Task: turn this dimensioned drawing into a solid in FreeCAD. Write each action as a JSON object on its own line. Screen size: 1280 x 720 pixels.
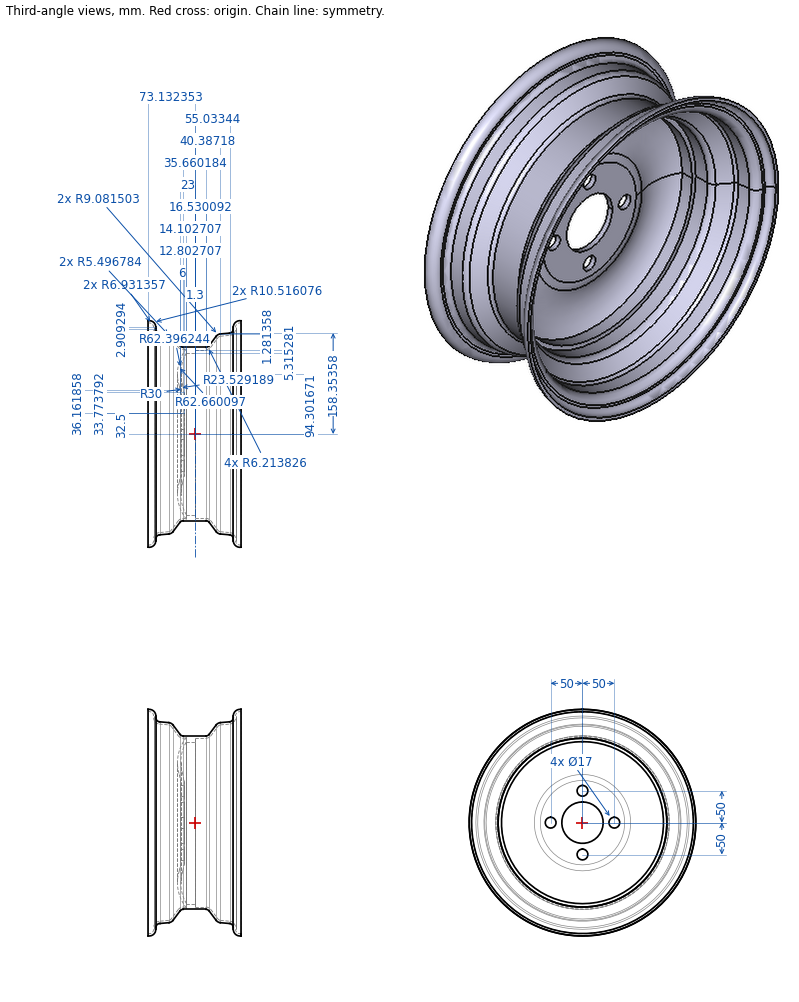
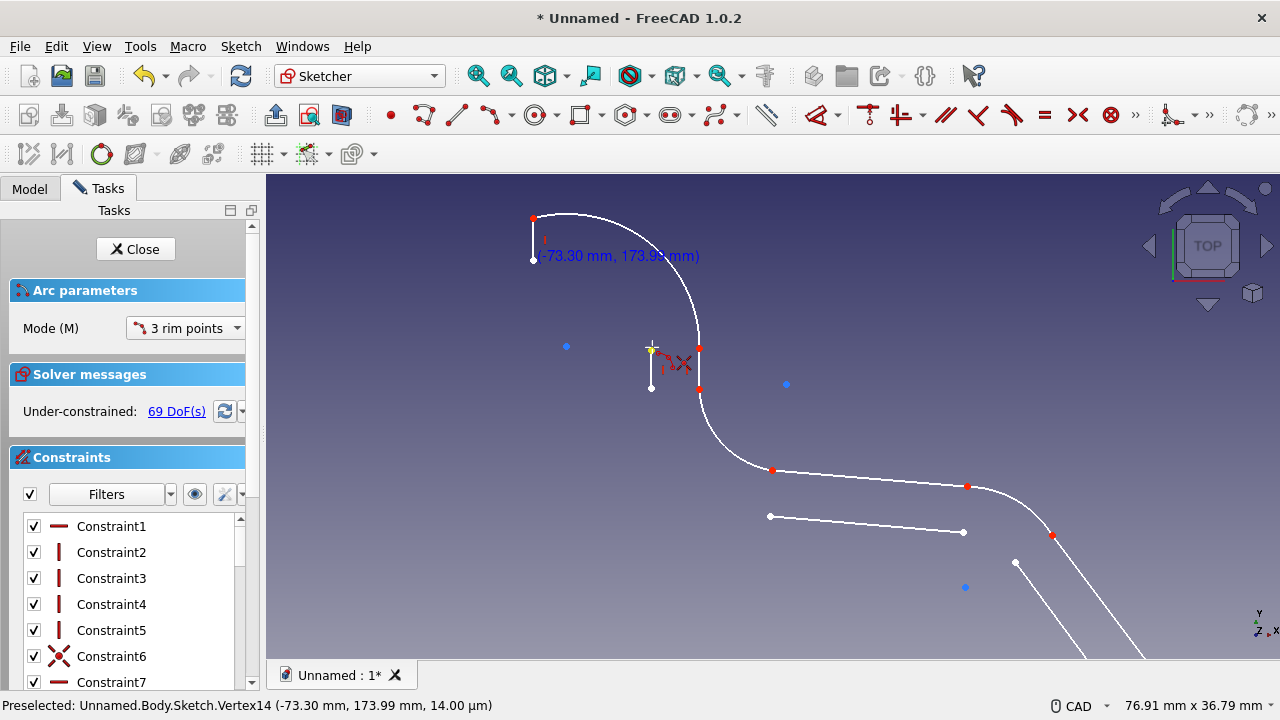
{"action": "left_click", "coordinate": [651, 351]}
{"action": "left_click", "coordinate": [615, 274]}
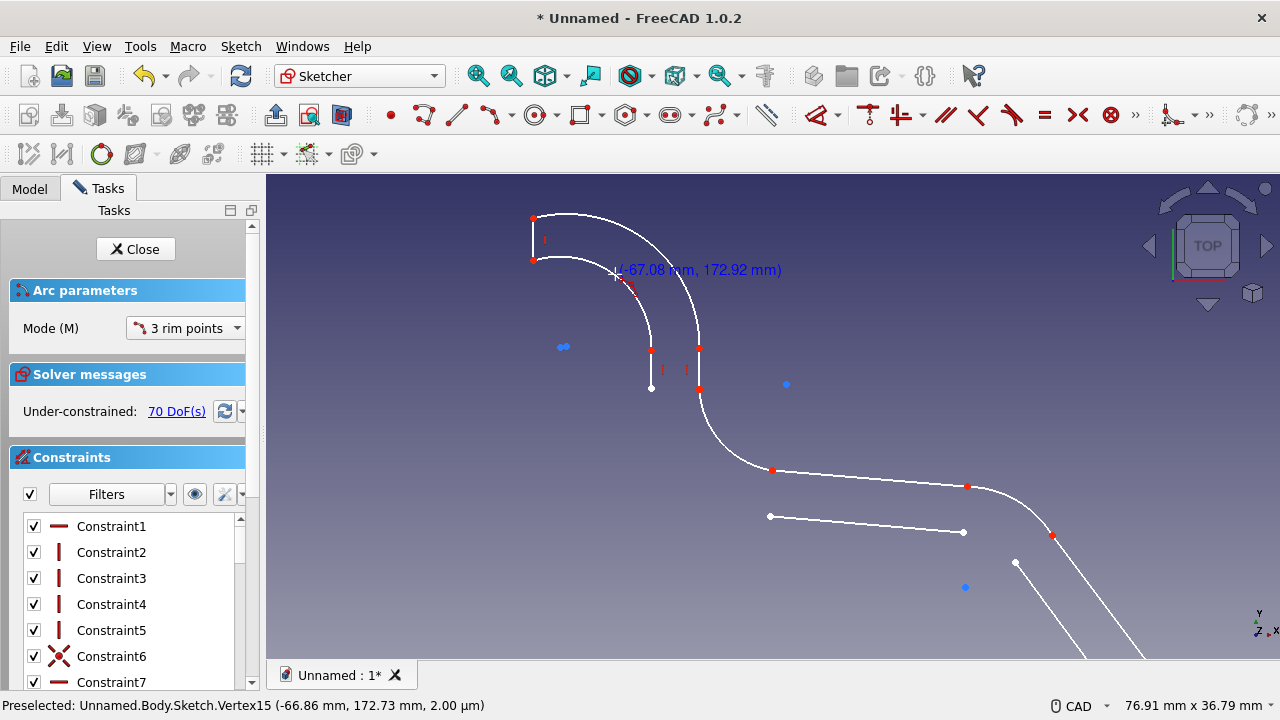
{"action": "left_click", "coordinate": [651, 389]}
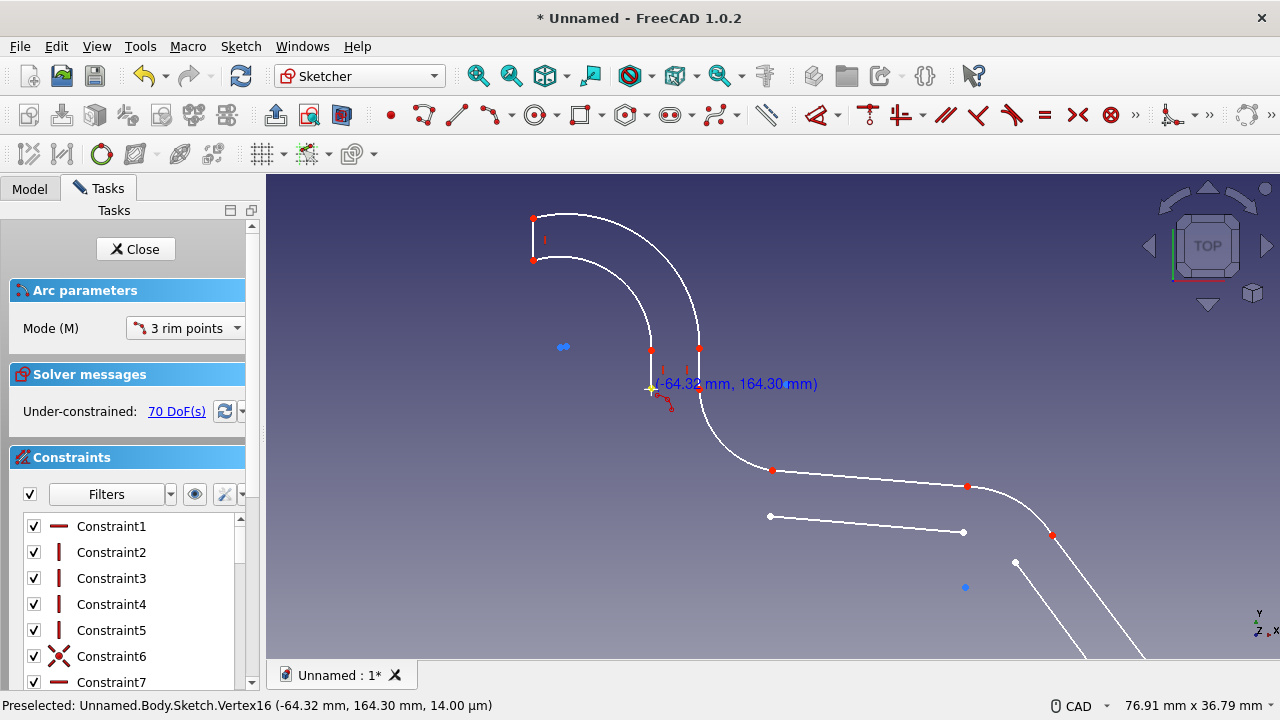
{"action": "scroll", "coordinate": [580, 265], "scroll_direction": "down", "scroll_amount": 10}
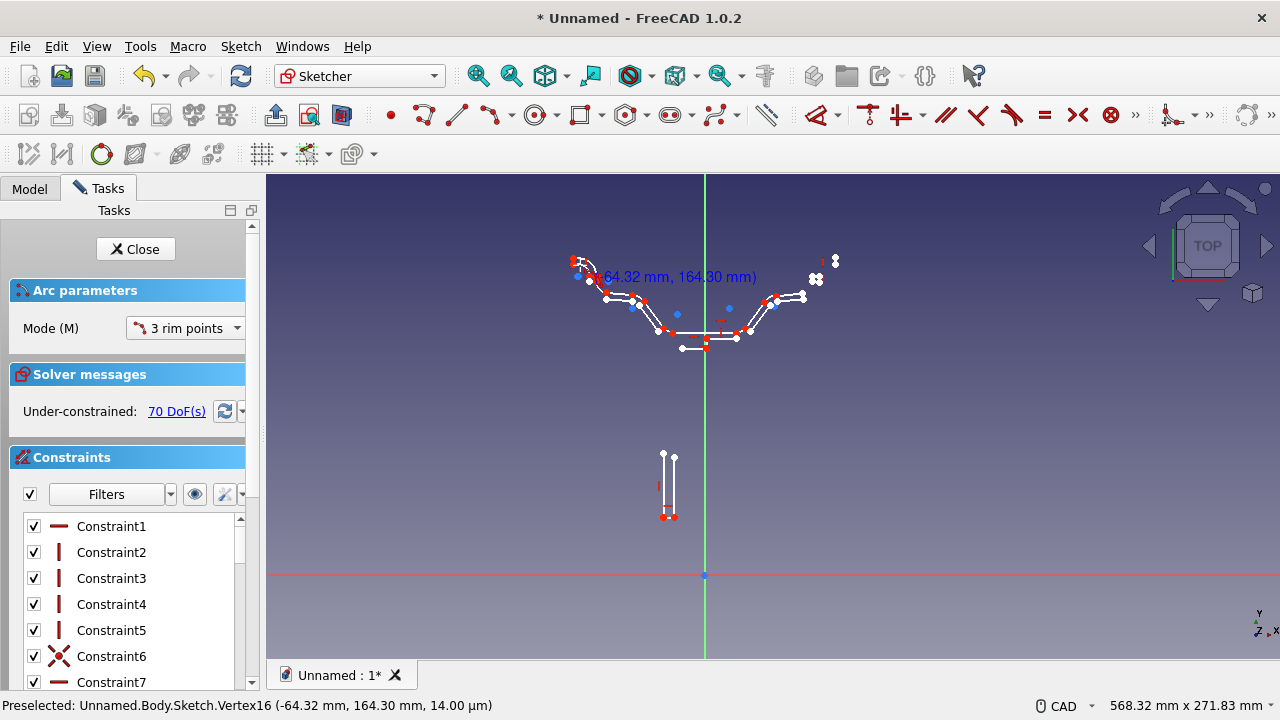
{"action": "scroll", "coordinate": [606, 299], "scroll_direction": "up", "scroll_amount": 5}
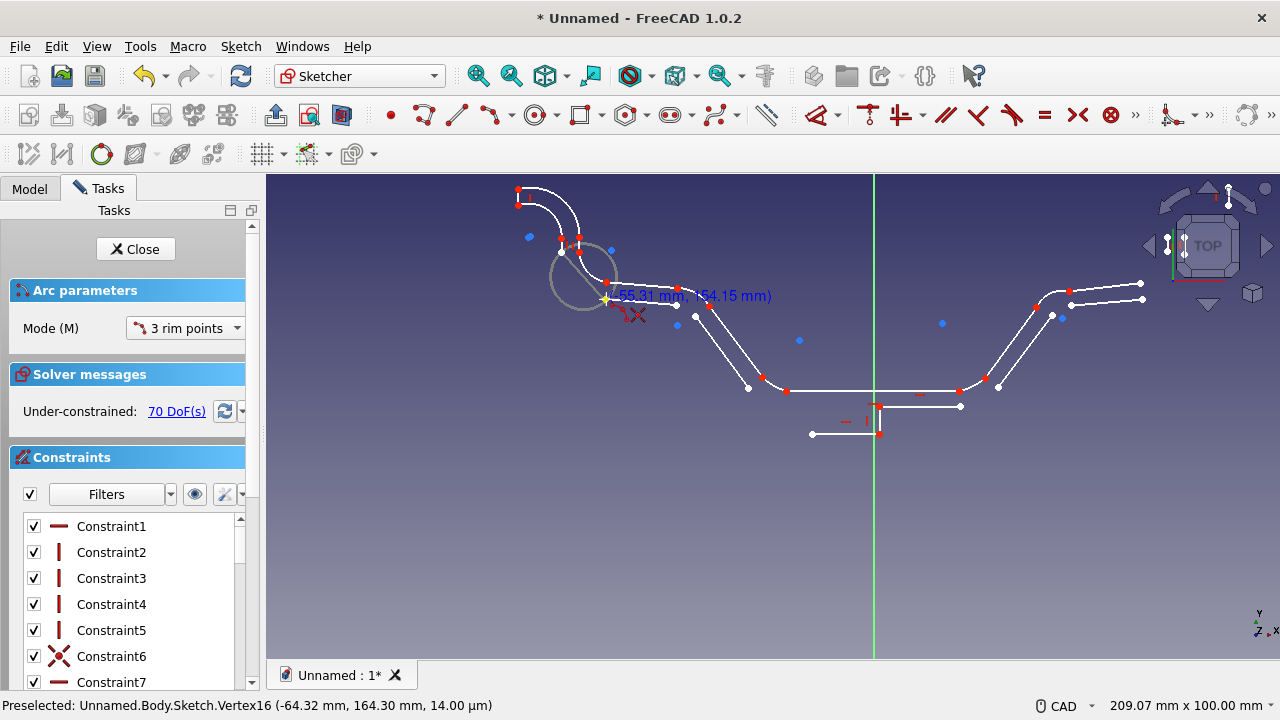
{"action": "left_click", "coordinate": [606, 299]}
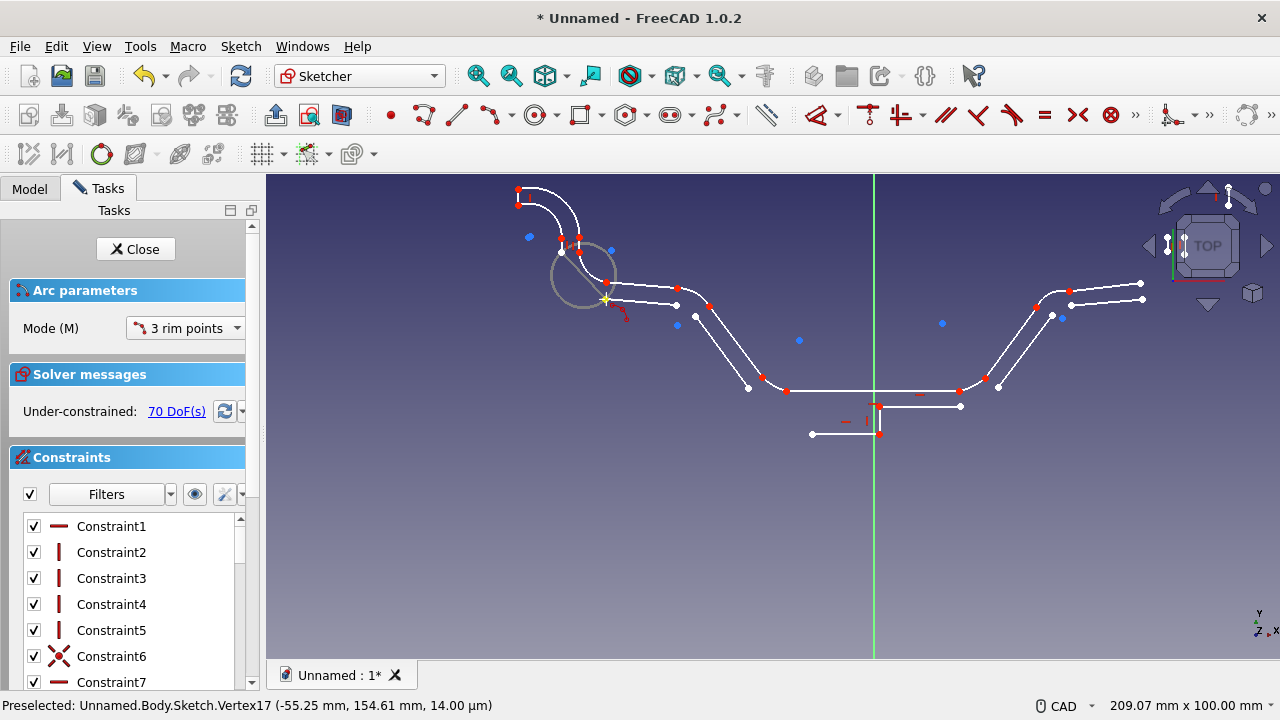
{"action": "scroll", "coordinate": [574, 283], "scroll_direction": "up", "scroll_amount": 2}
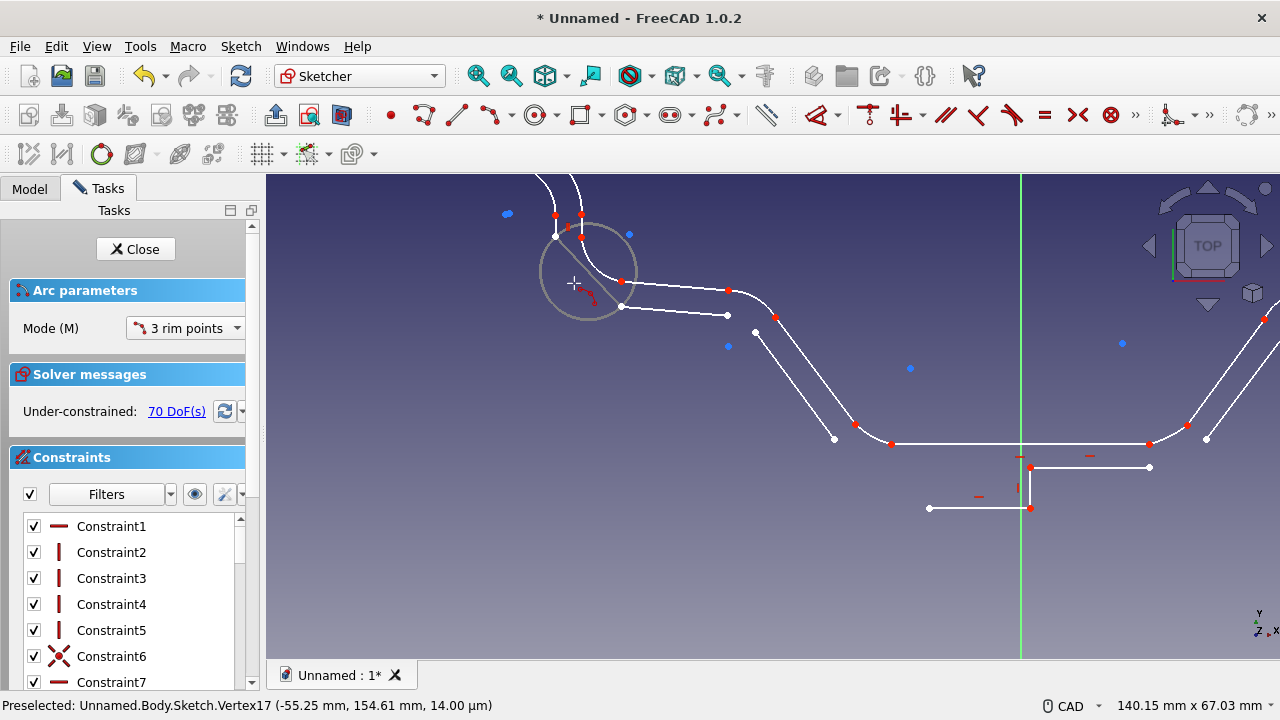
{"action": "left_click", "coordinate": [574, 283]}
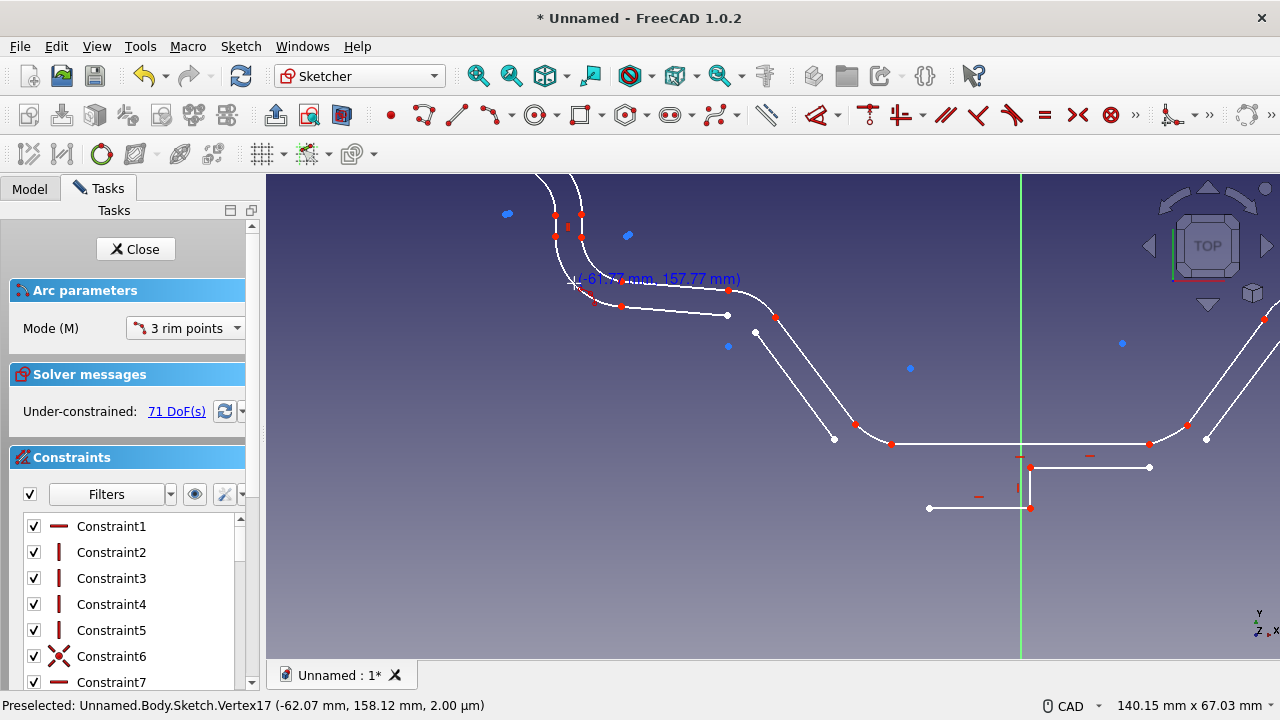
{"action": "left_click", "coordinate": [727, 316]}
{"action": "left_click", "coordinate": [755, 332]}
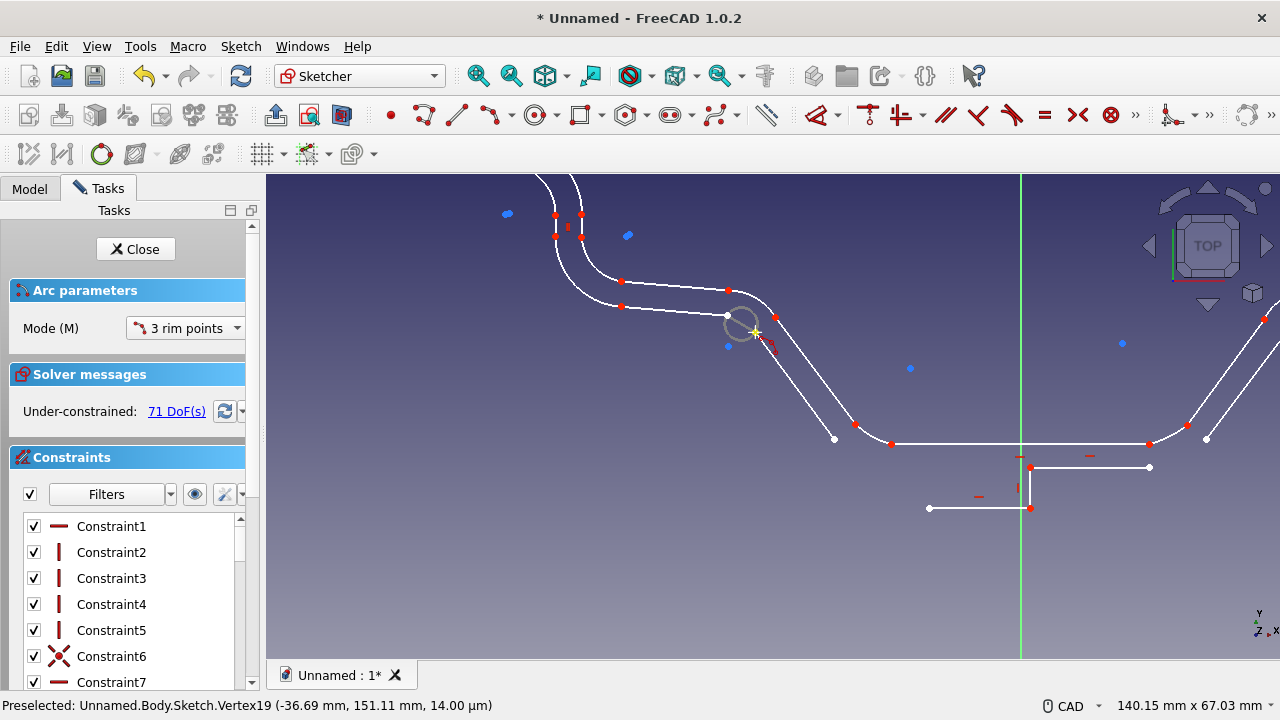
{"action": "scroll", "coordinate": [742, 320], "scroll_direction": "up", "scroll_amount": 8}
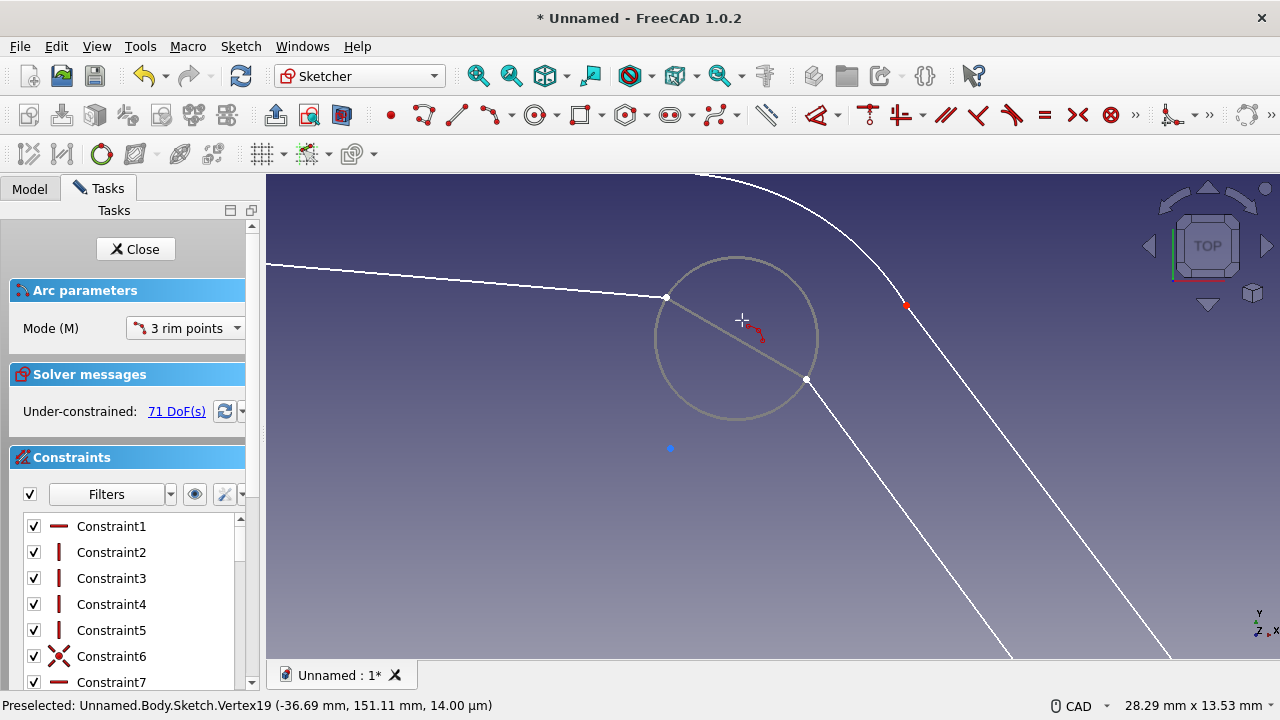
{"action": "left_click", "coordinate": [742, 318]}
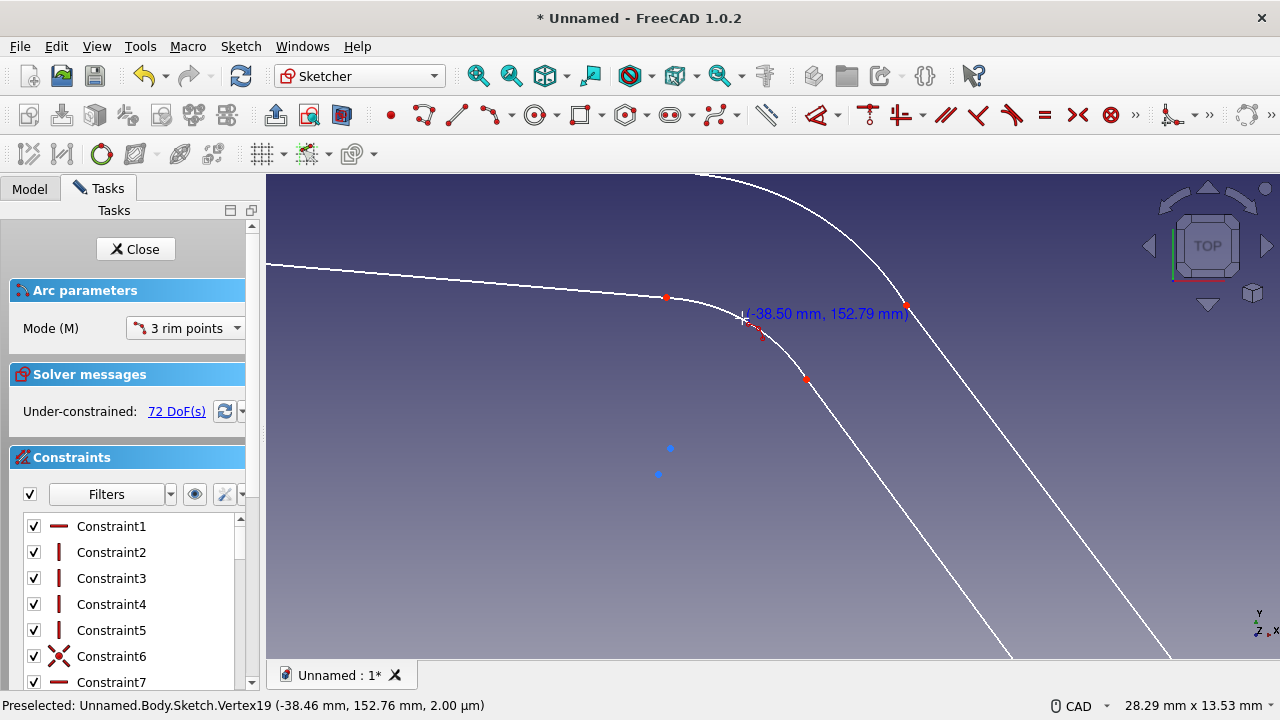
{"action": "scroll", "coordinate": [630, 302], "scroll_direction": "down", "scroll_amount": 15}